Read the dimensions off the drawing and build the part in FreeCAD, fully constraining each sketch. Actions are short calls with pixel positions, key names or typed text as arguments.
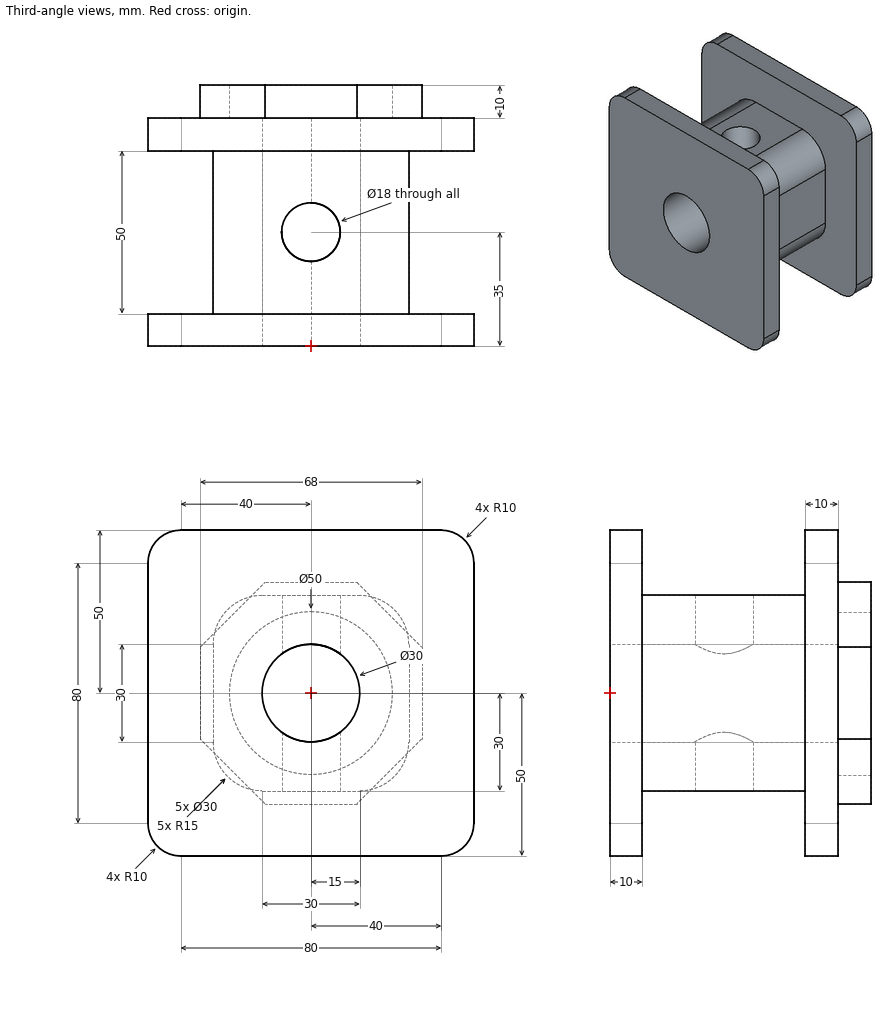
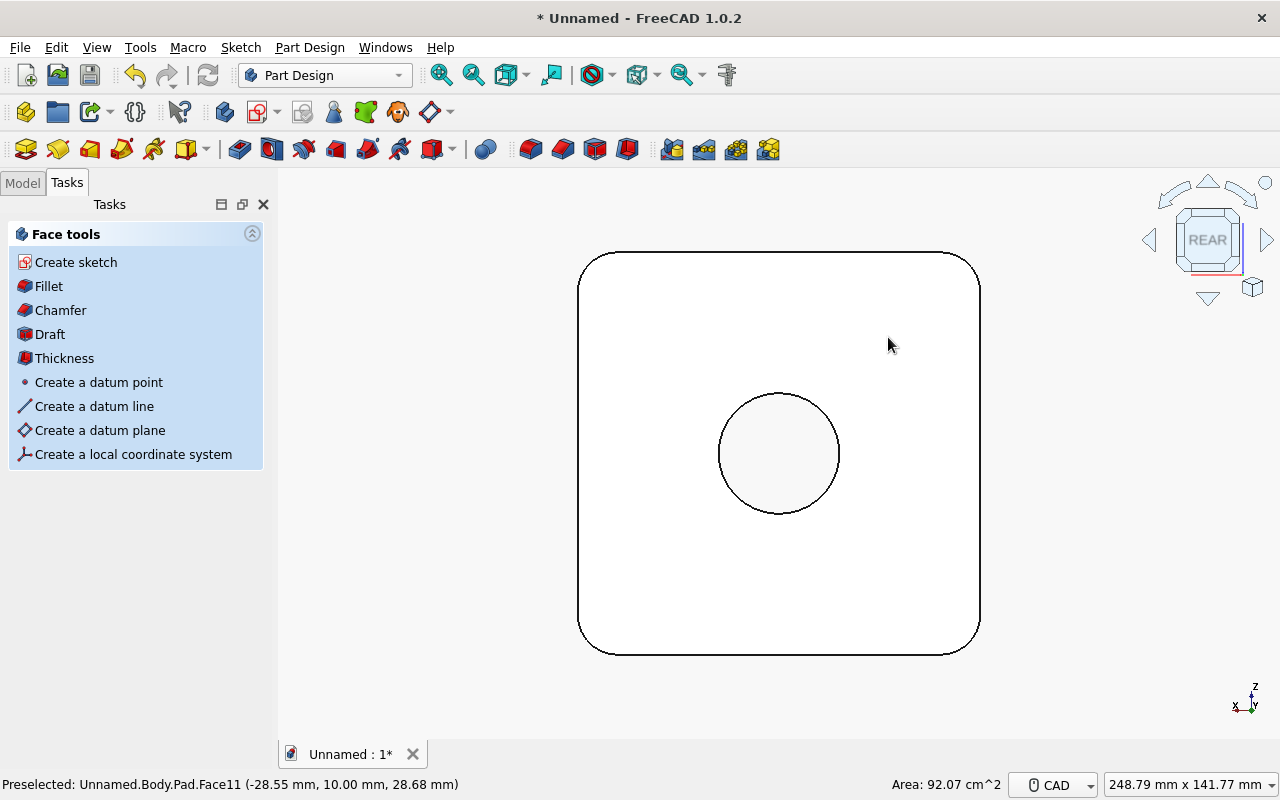
click(258, 112)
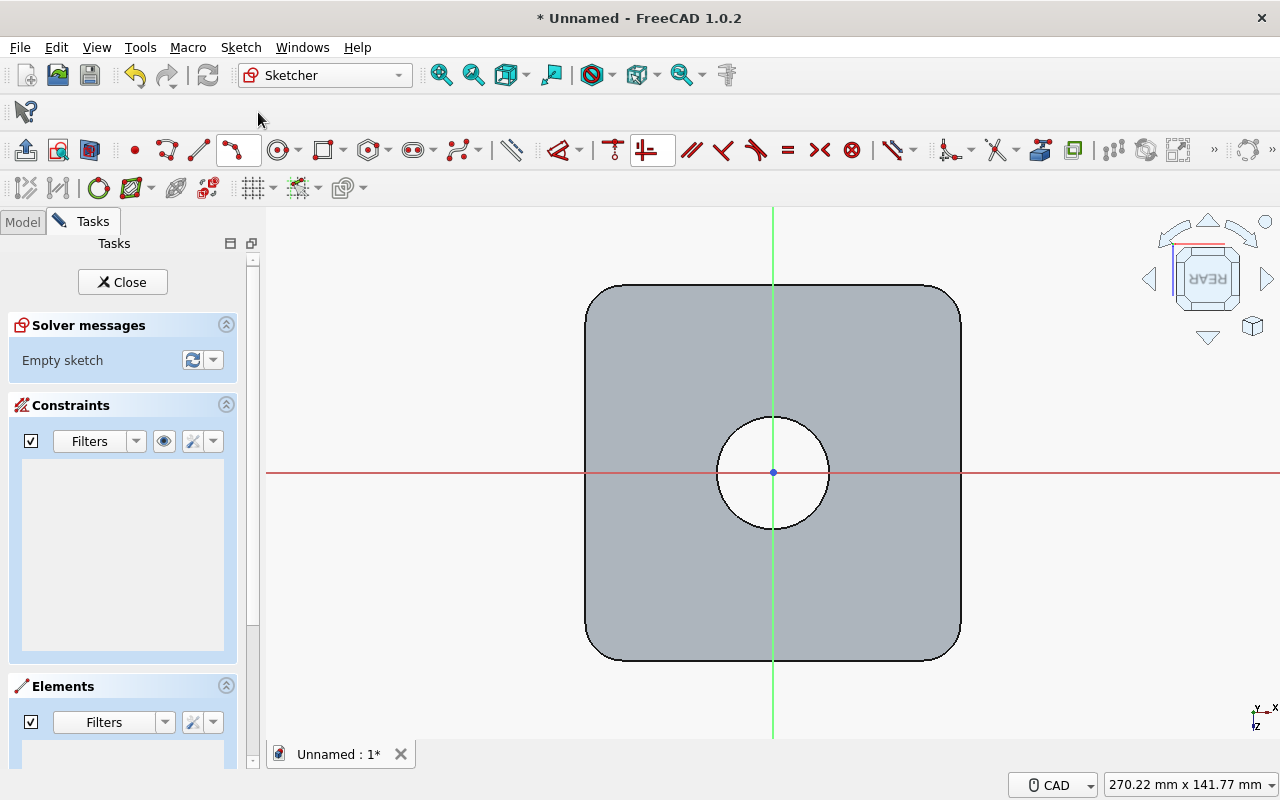
scroll(912, 473, up, 2)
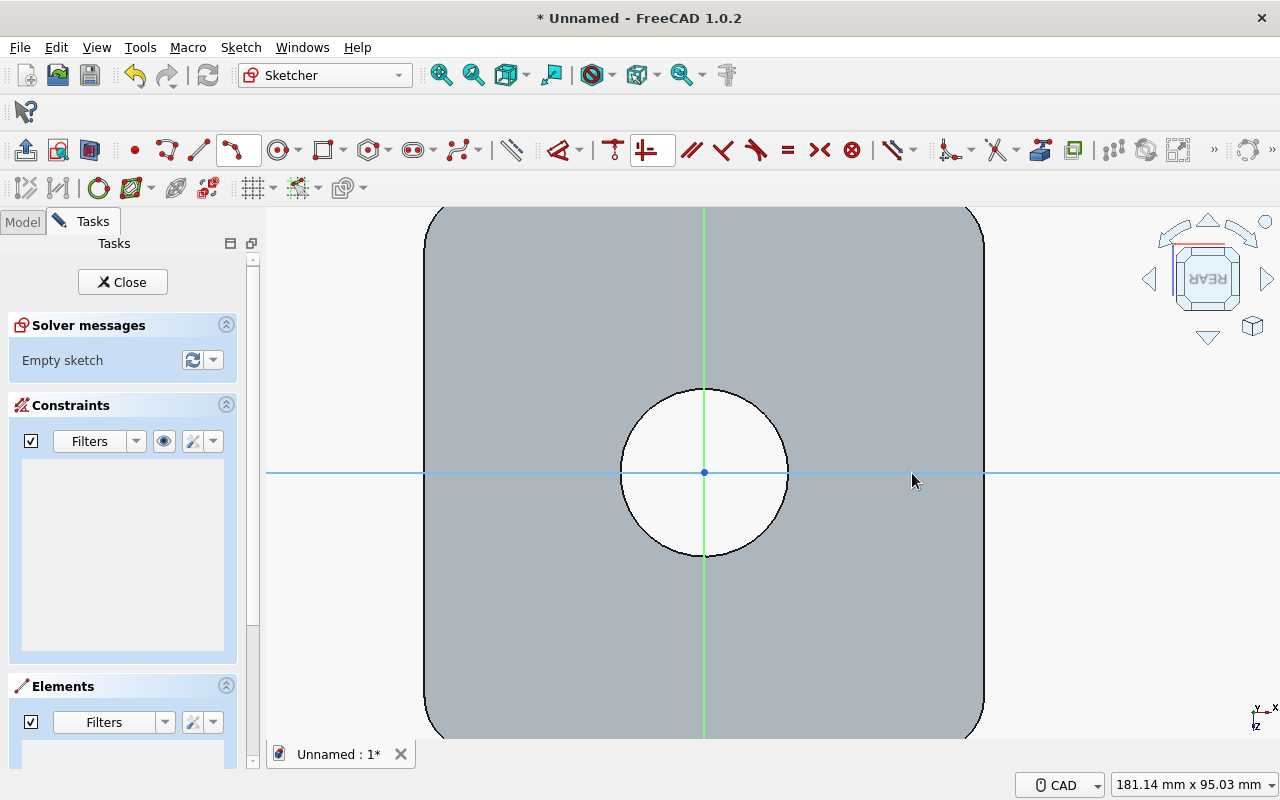
click(200, 150)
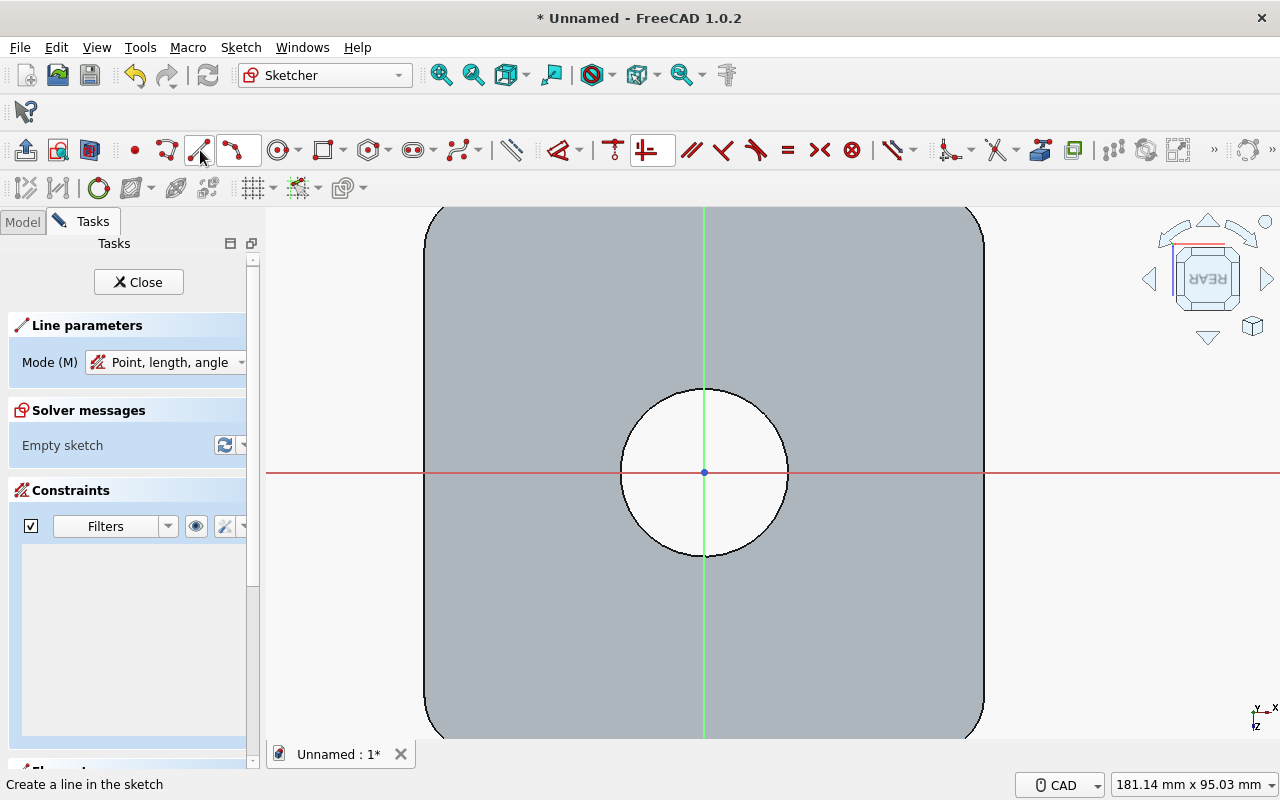
click(788, 305)
click(620, 305)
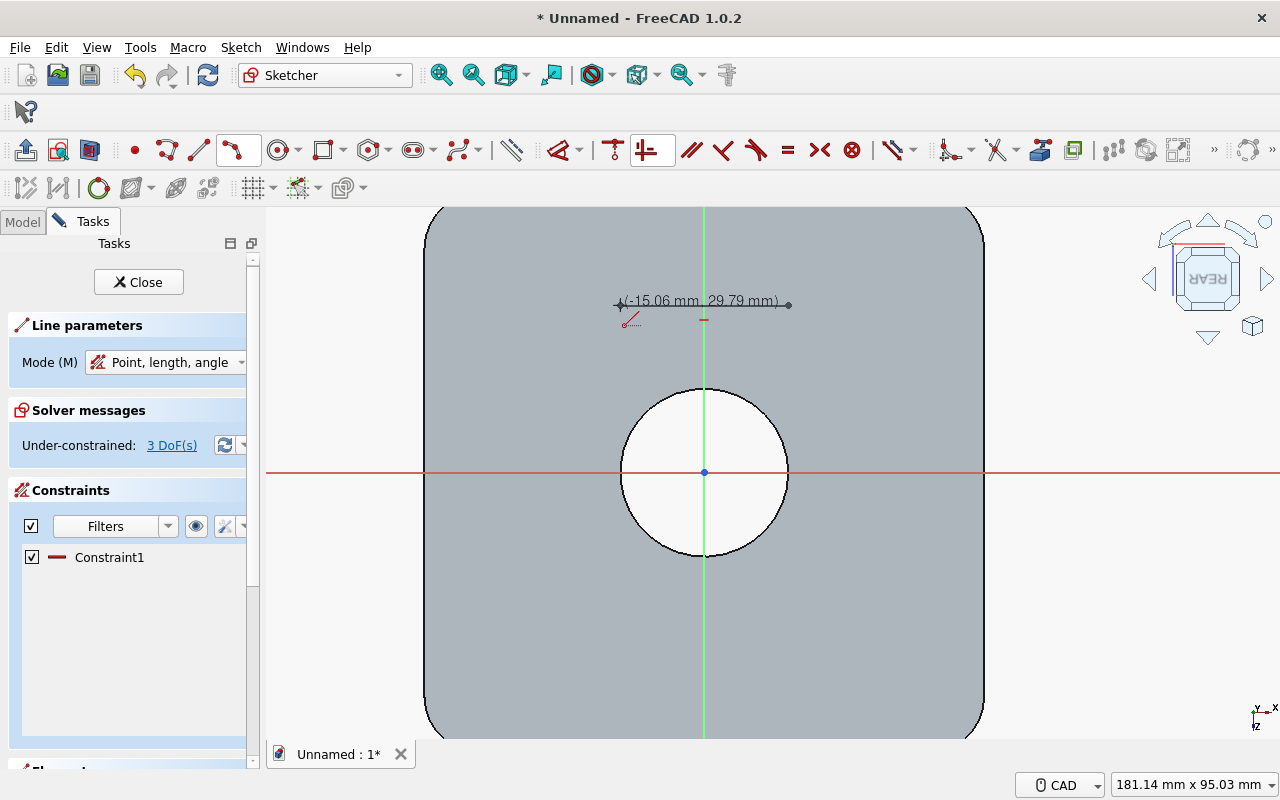
click(536, 389)
click(536, 557)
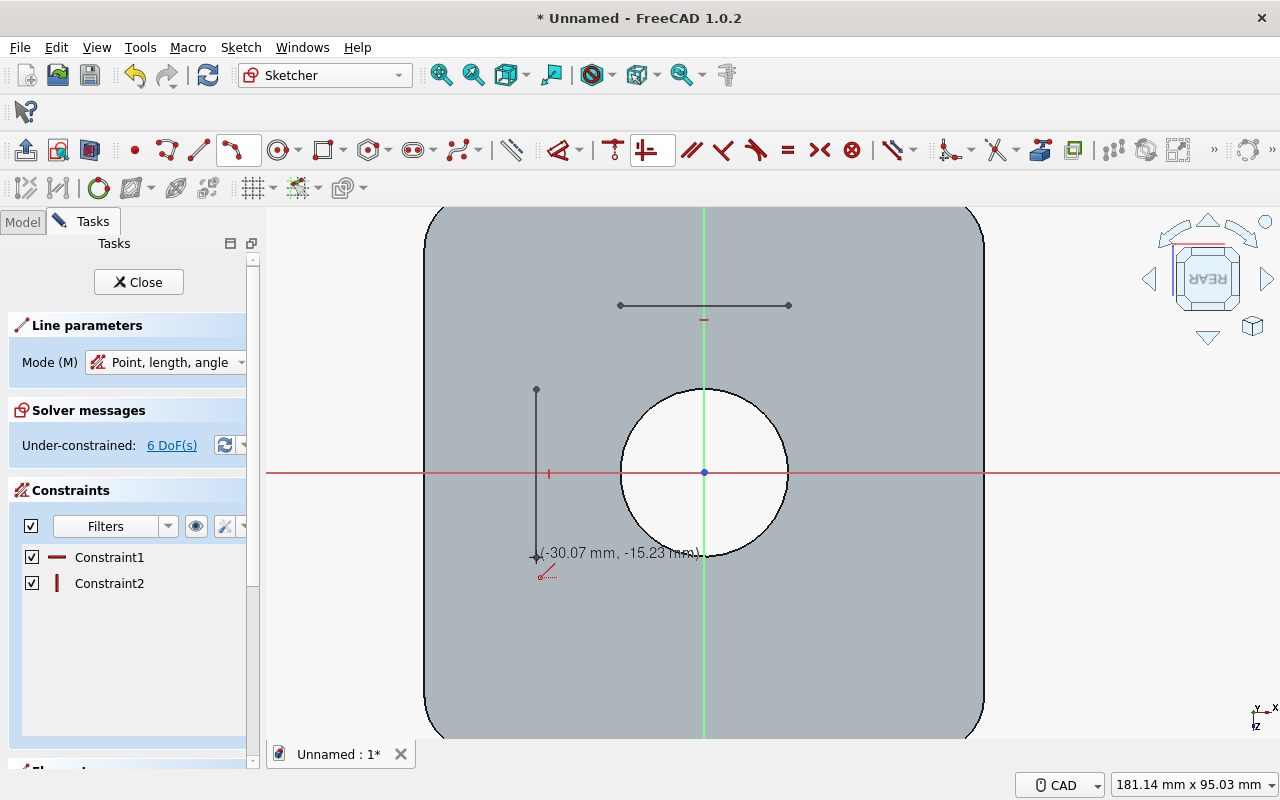
click(620, 641)
click(788, 641)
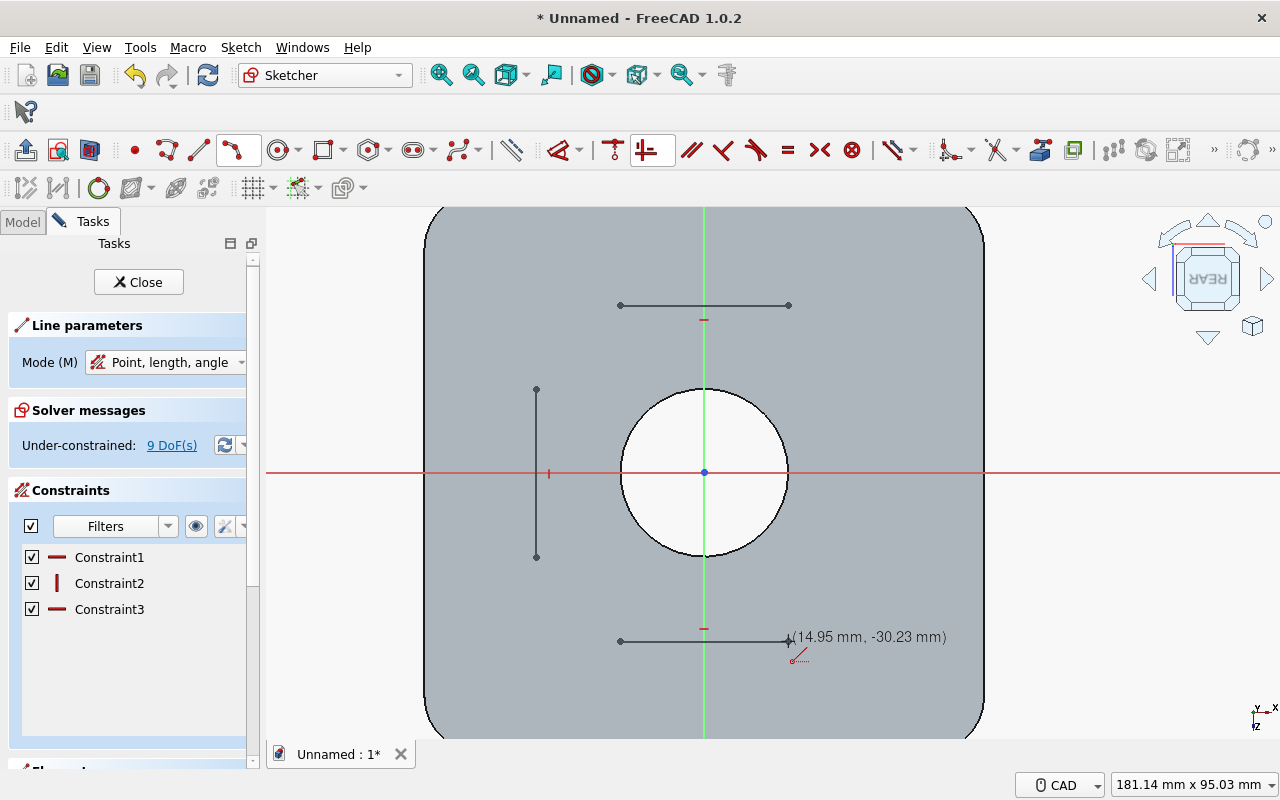
click(872, 557)
click(872, 389)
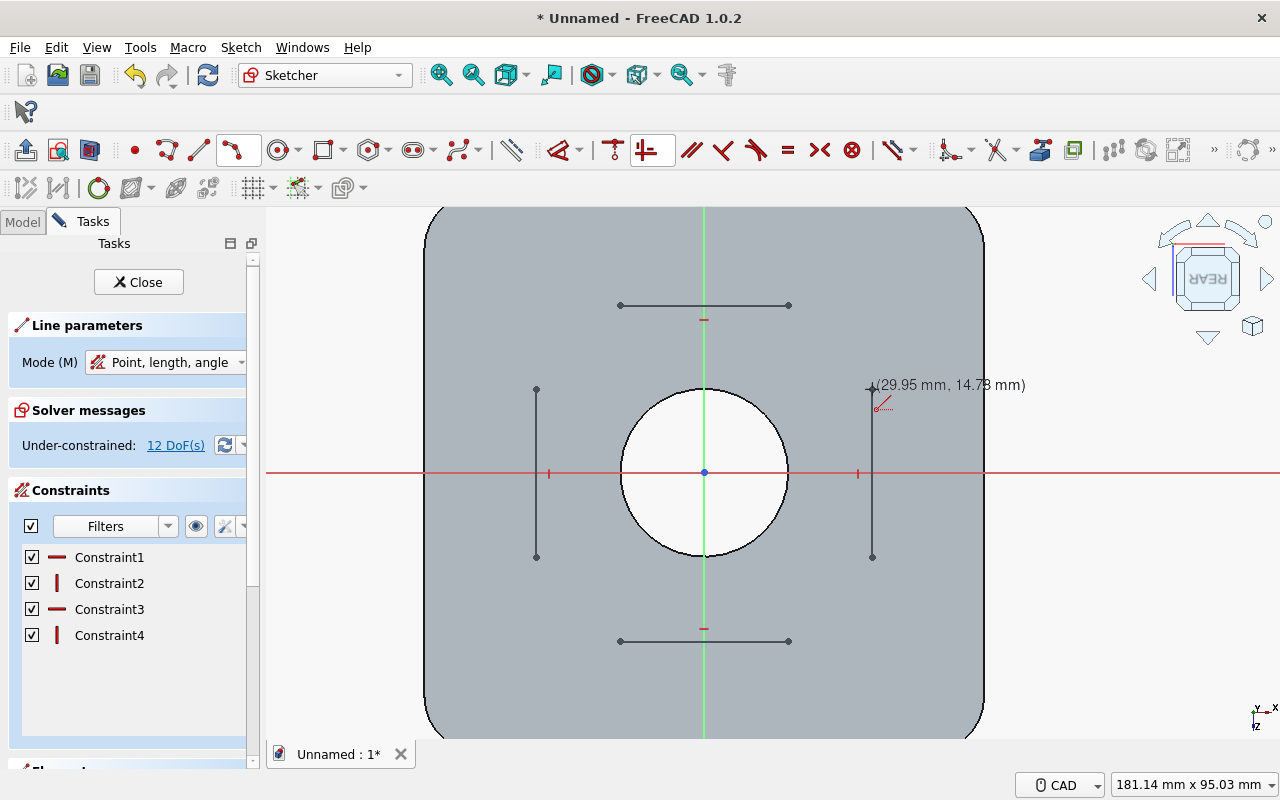
click(232, 150)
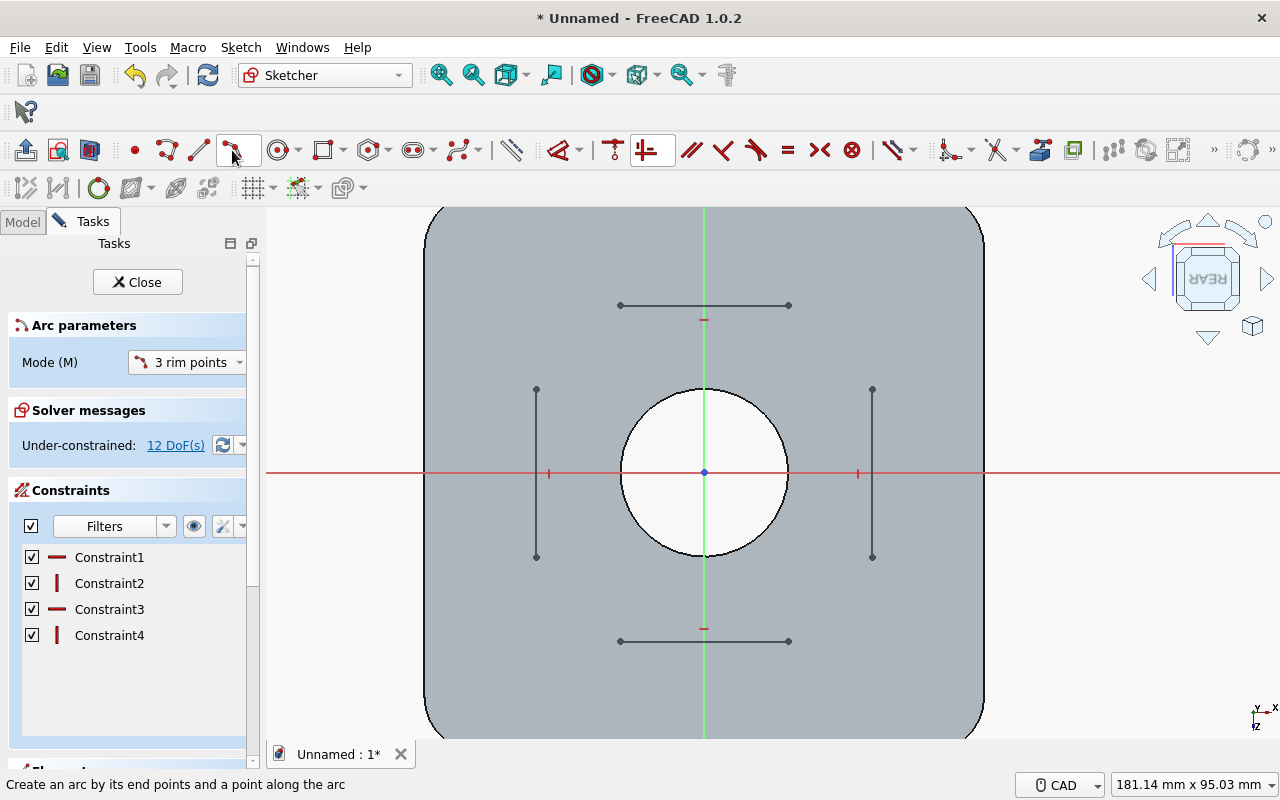
click(620, 306)
click(536, 390)
click(561, 329)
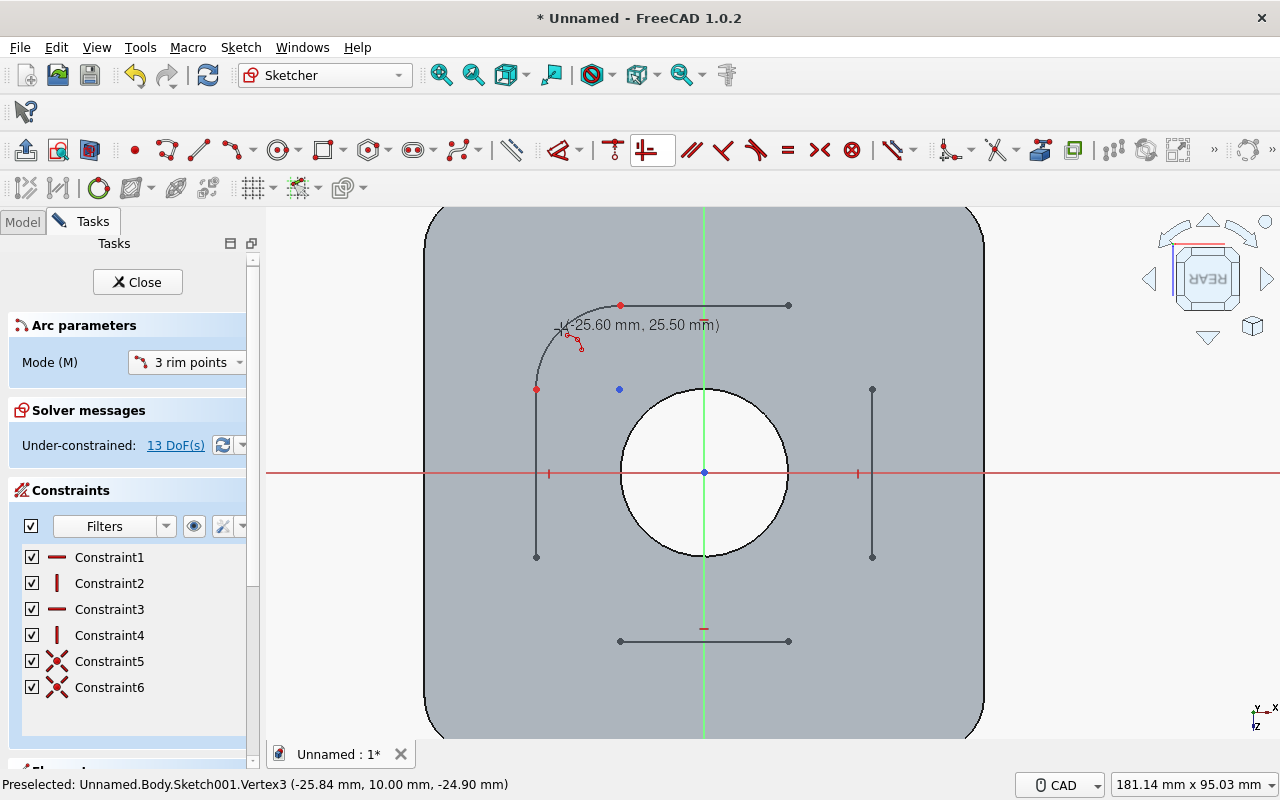
click(536, 558)
click(620, 642)
click(561, 616)